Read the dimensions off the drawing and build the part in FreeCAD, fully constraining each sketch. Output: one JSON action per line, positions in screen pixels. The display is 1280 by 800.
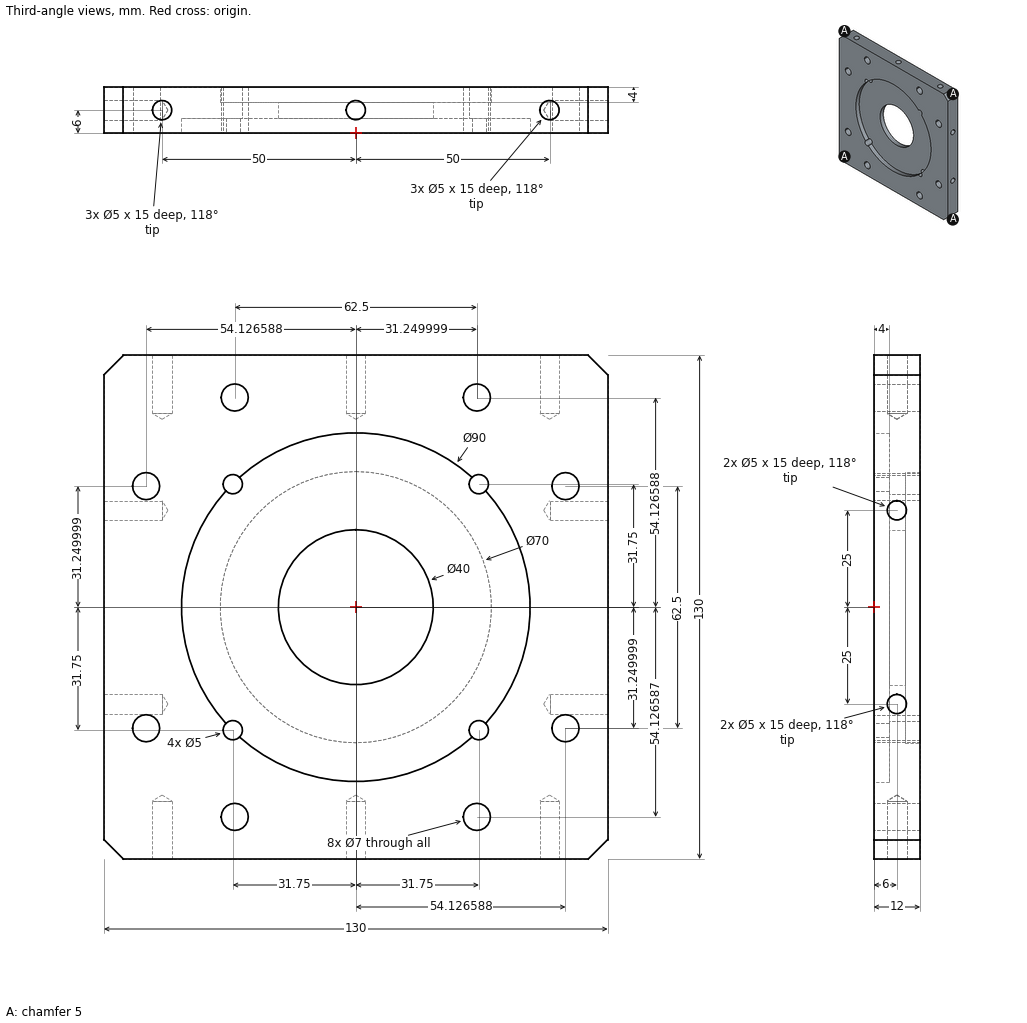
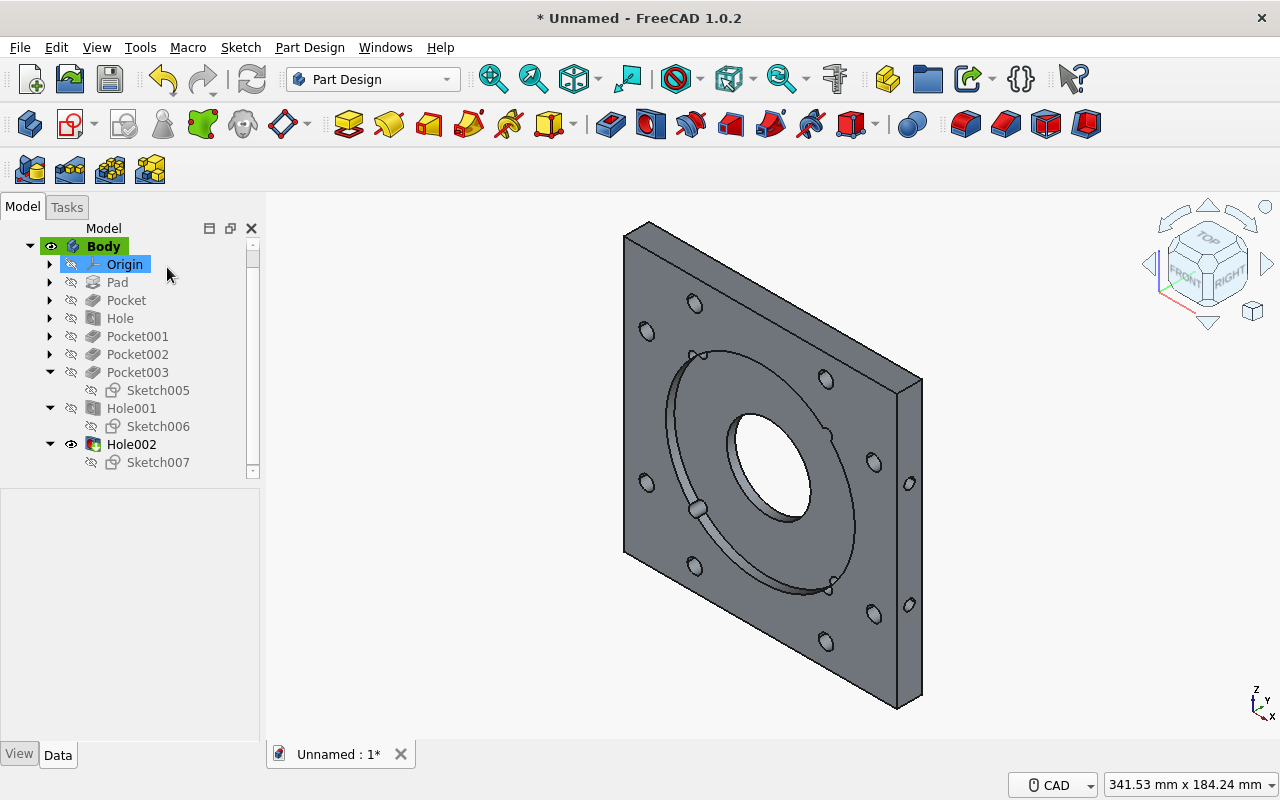
{"action": "left_click", "coordinate": [890, 374]}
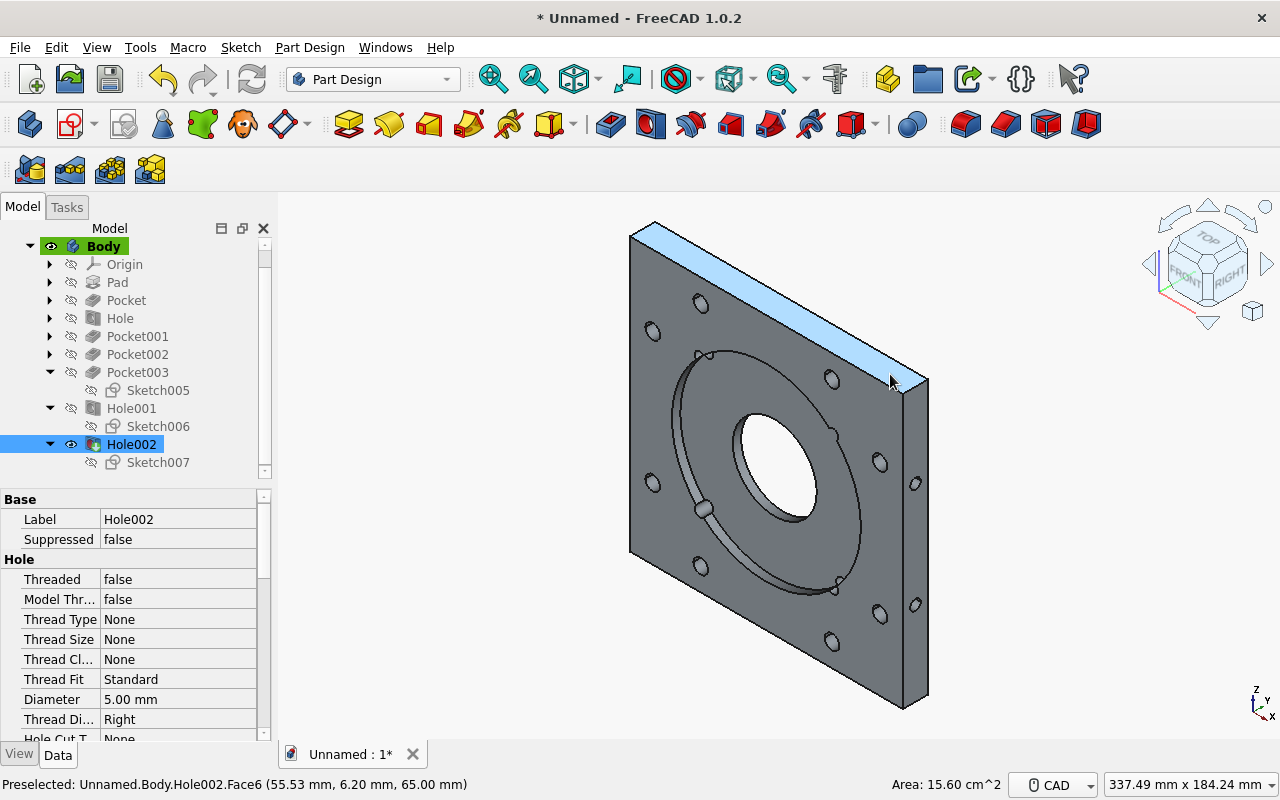
{"action": "left_click", "coordinate": [70, 124]}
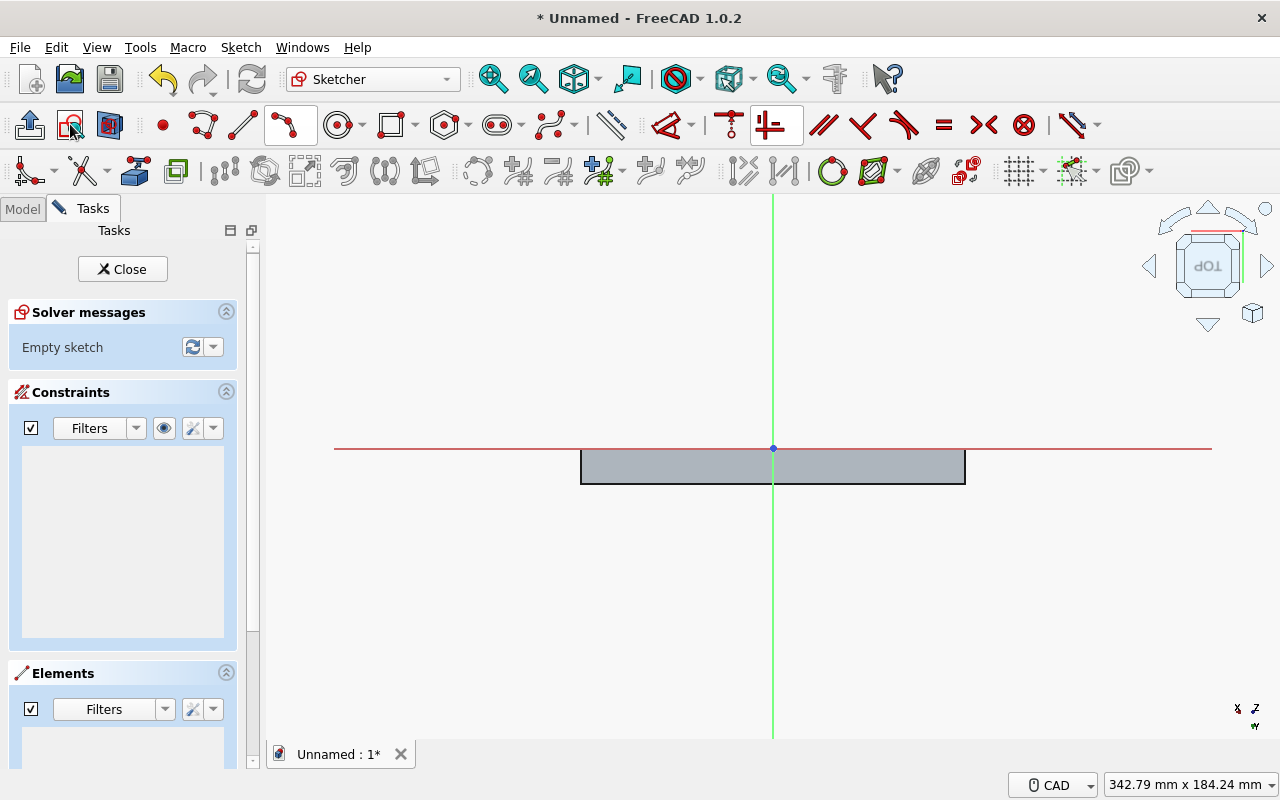
{"action": "scroll", "coordinate": [856, 455], "scroll_direction": "up", "scroll_amount": 3}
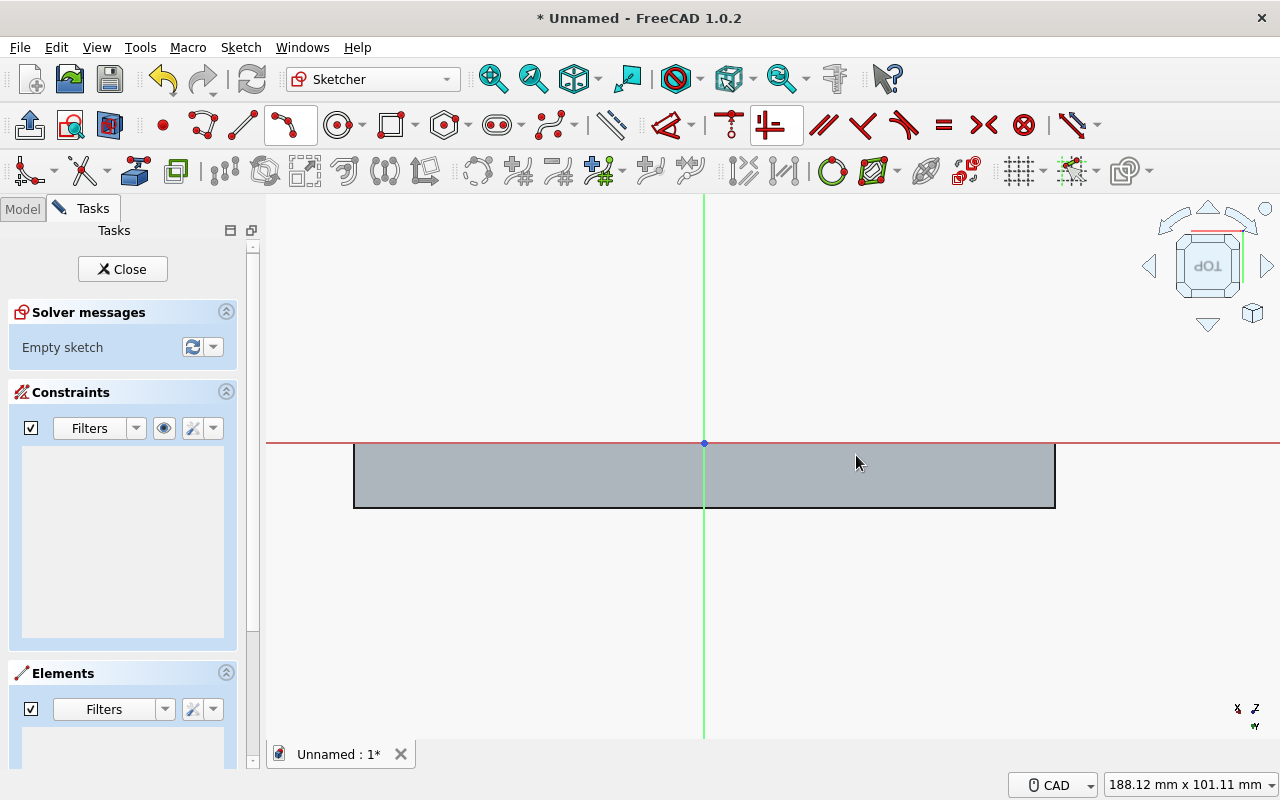
{"action": "key", "text": "g c"}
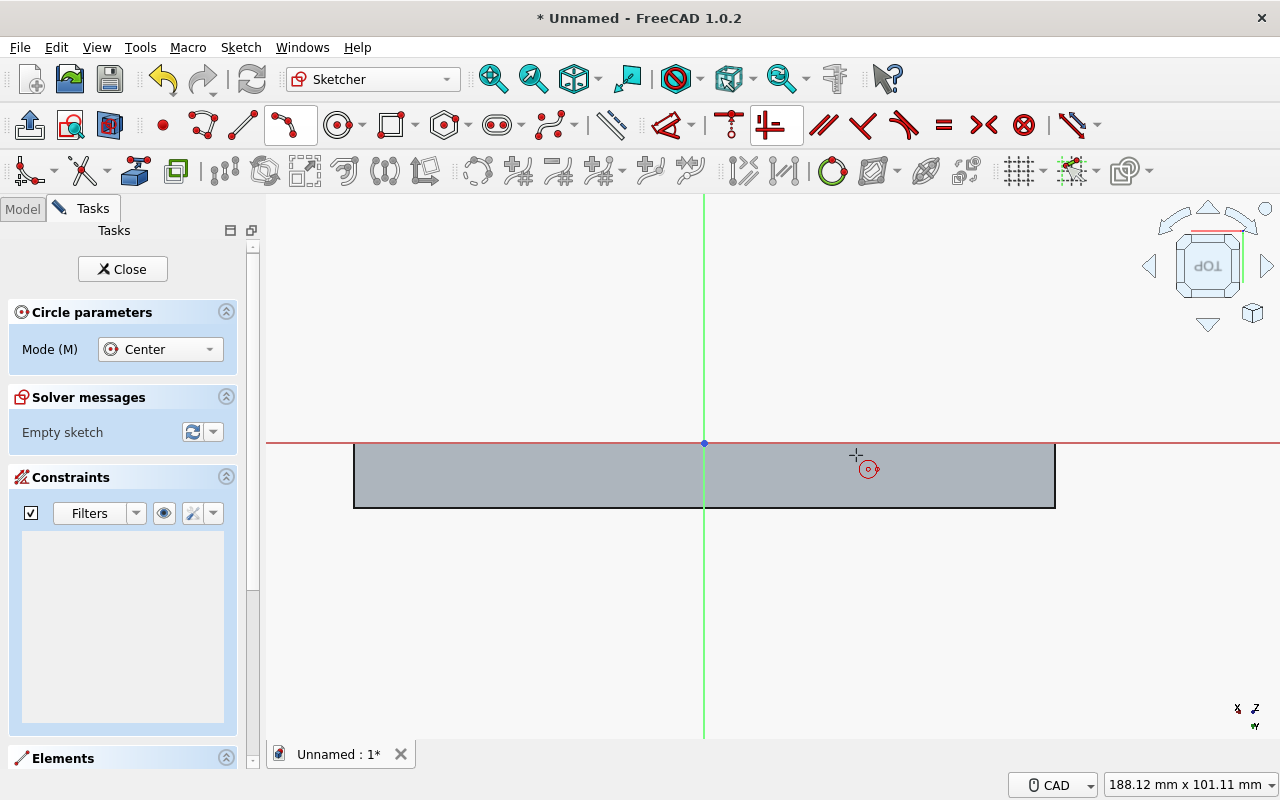
{"action": "scroll", "coordinate": [974, 476], "scroll_direction": "up", "scroll_amount": 3}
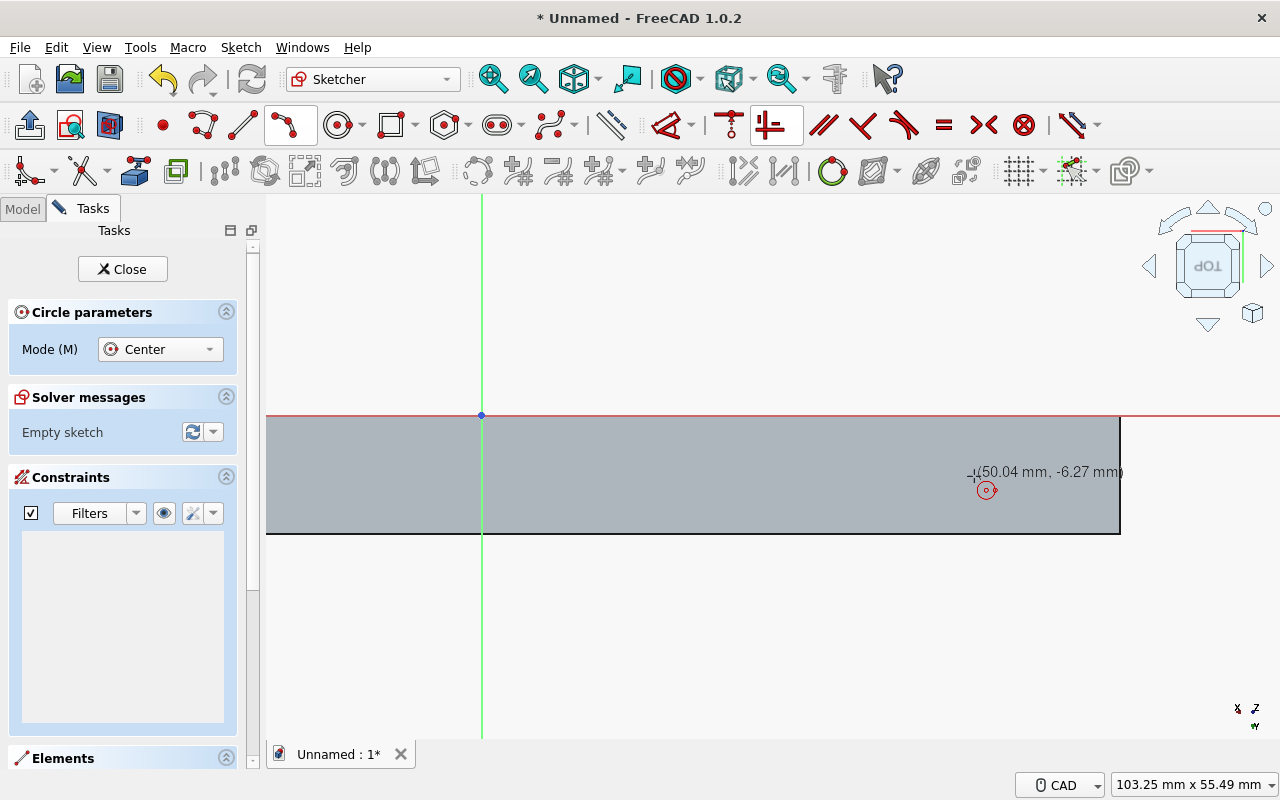
{"action": "left_click", "coordinate": [973, 475]}
{"action": "left_click", "coordinate": [990, 457]}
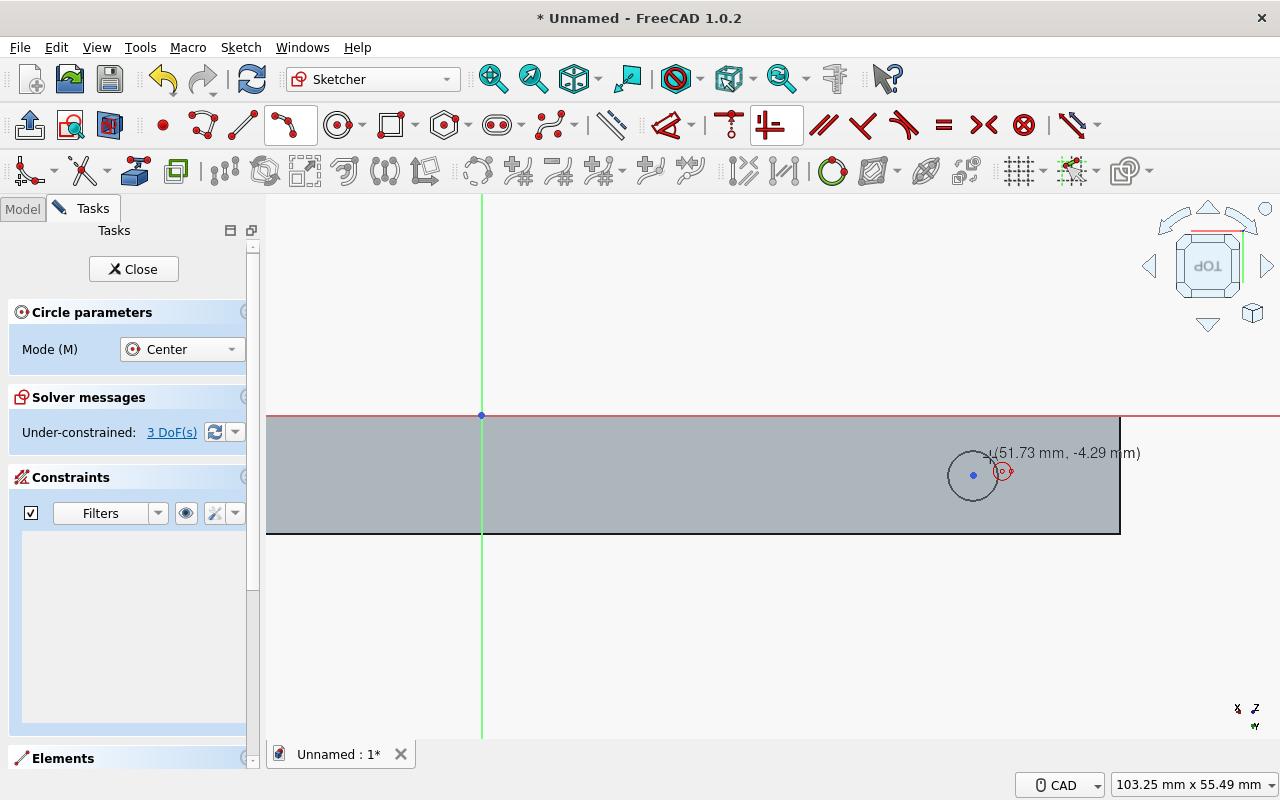
{"action": "scroll", "coordinate": [975, 477], "scroll_direction": "down", "scroll_amount": 3}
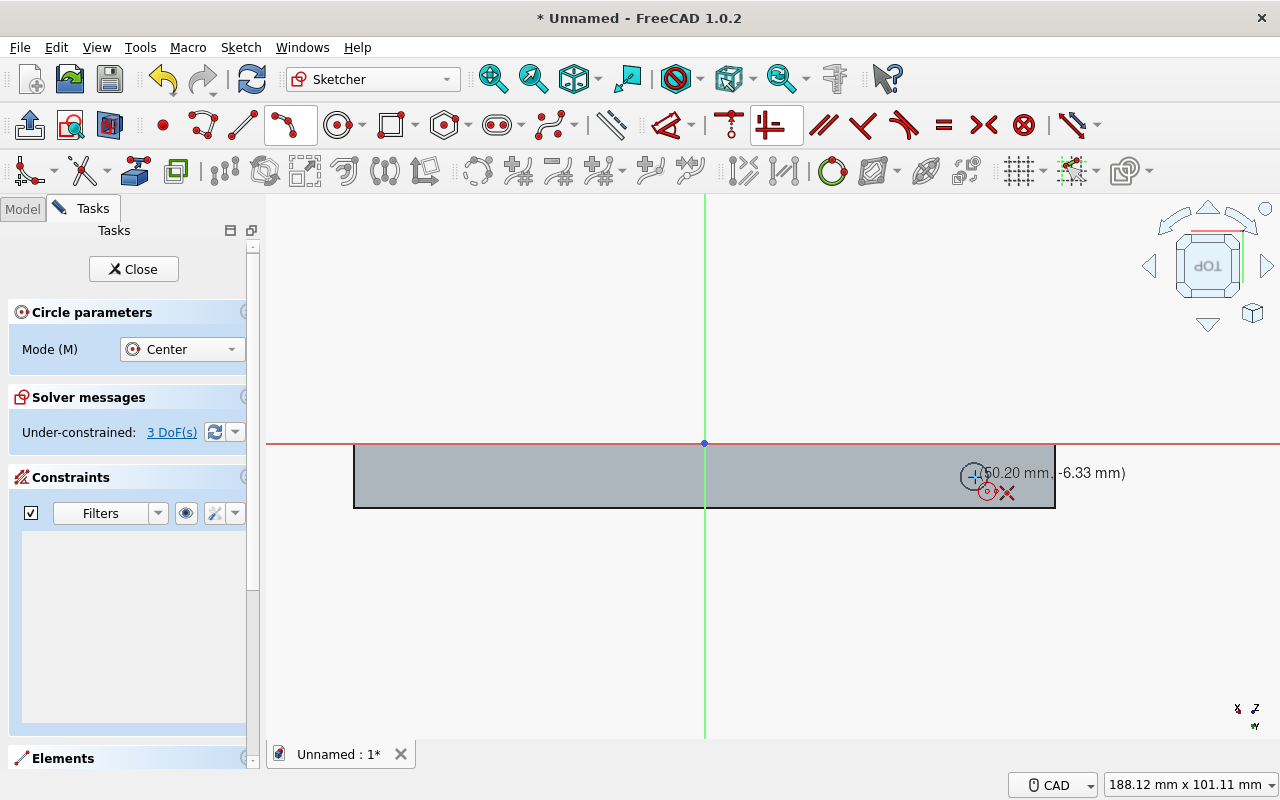
{"action": "scroll", "coordinate": [435, 476], "scroll_direction": "up", "scroll_amount": 3}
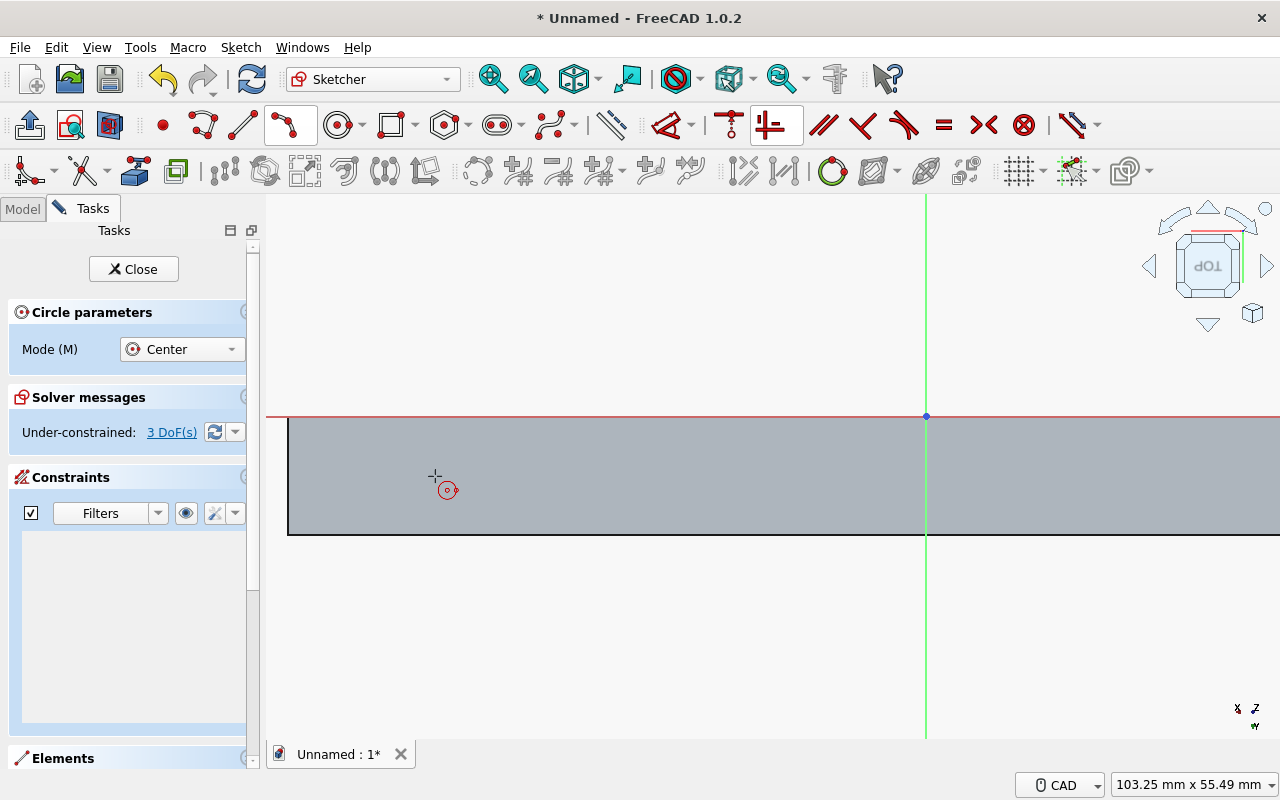
{"action": "left_click", "coordinate": [435, 476]}
{"action": "left_click", "coordinate": [453, 458]}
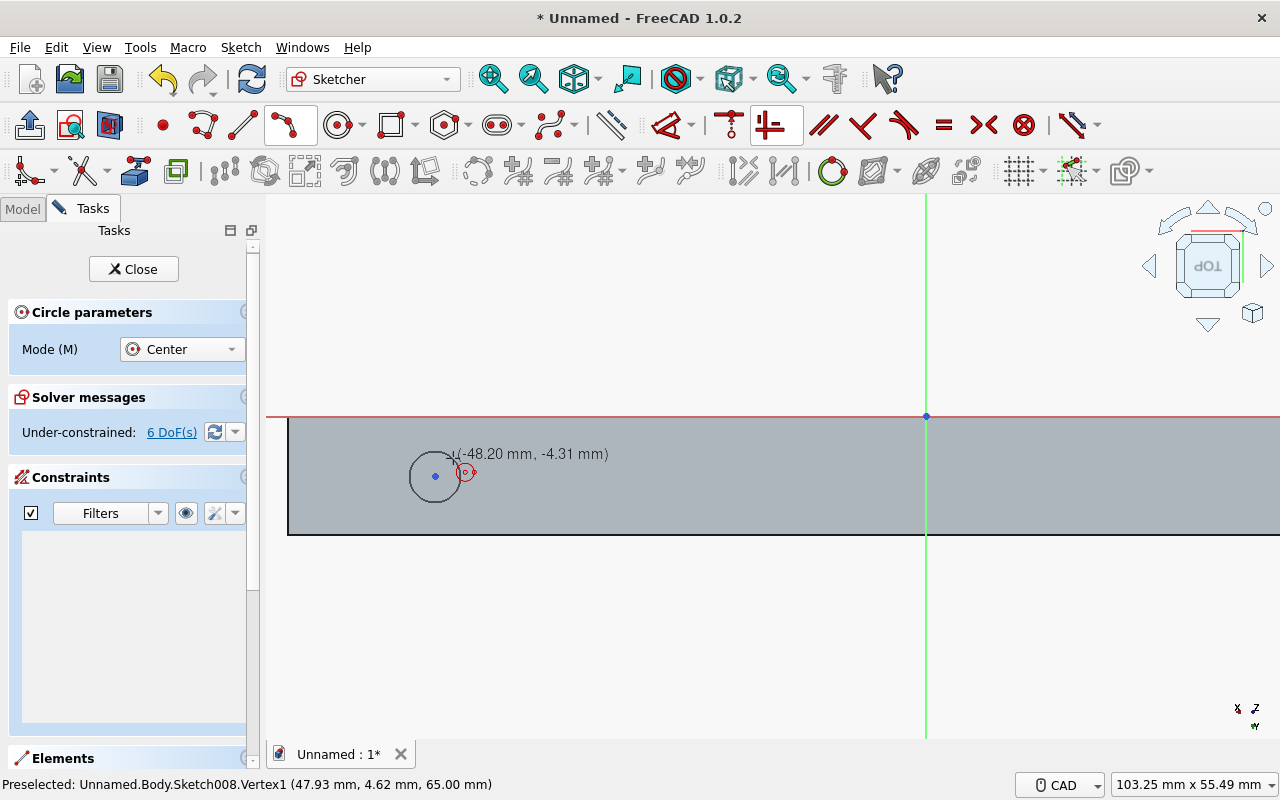
{"action": "left_click", "coordinate": [926, 476]}
{"action": "left_click", "coordinate": [944, 458]}
{"action": "key", "text": "Escape"}